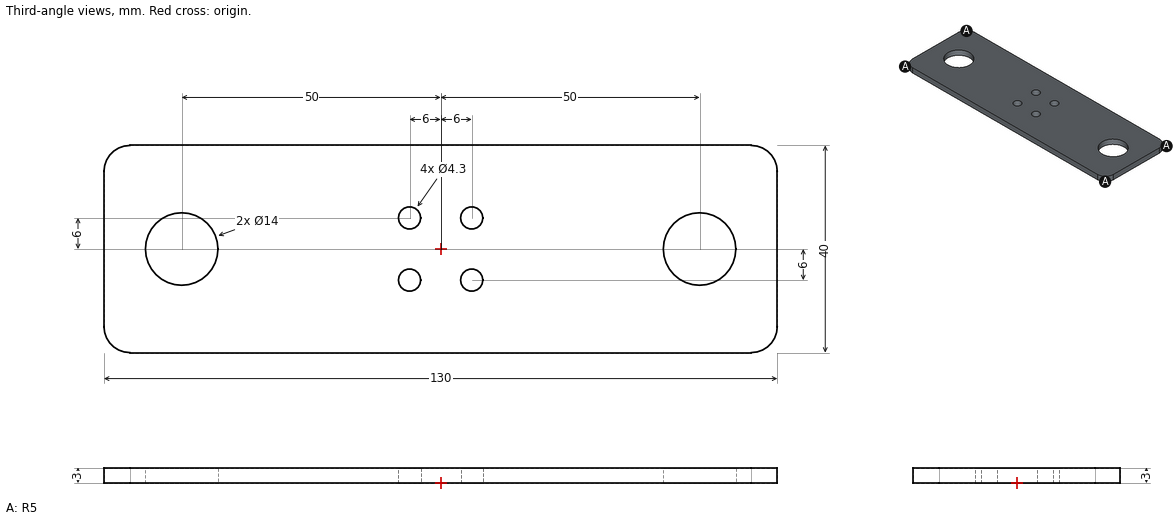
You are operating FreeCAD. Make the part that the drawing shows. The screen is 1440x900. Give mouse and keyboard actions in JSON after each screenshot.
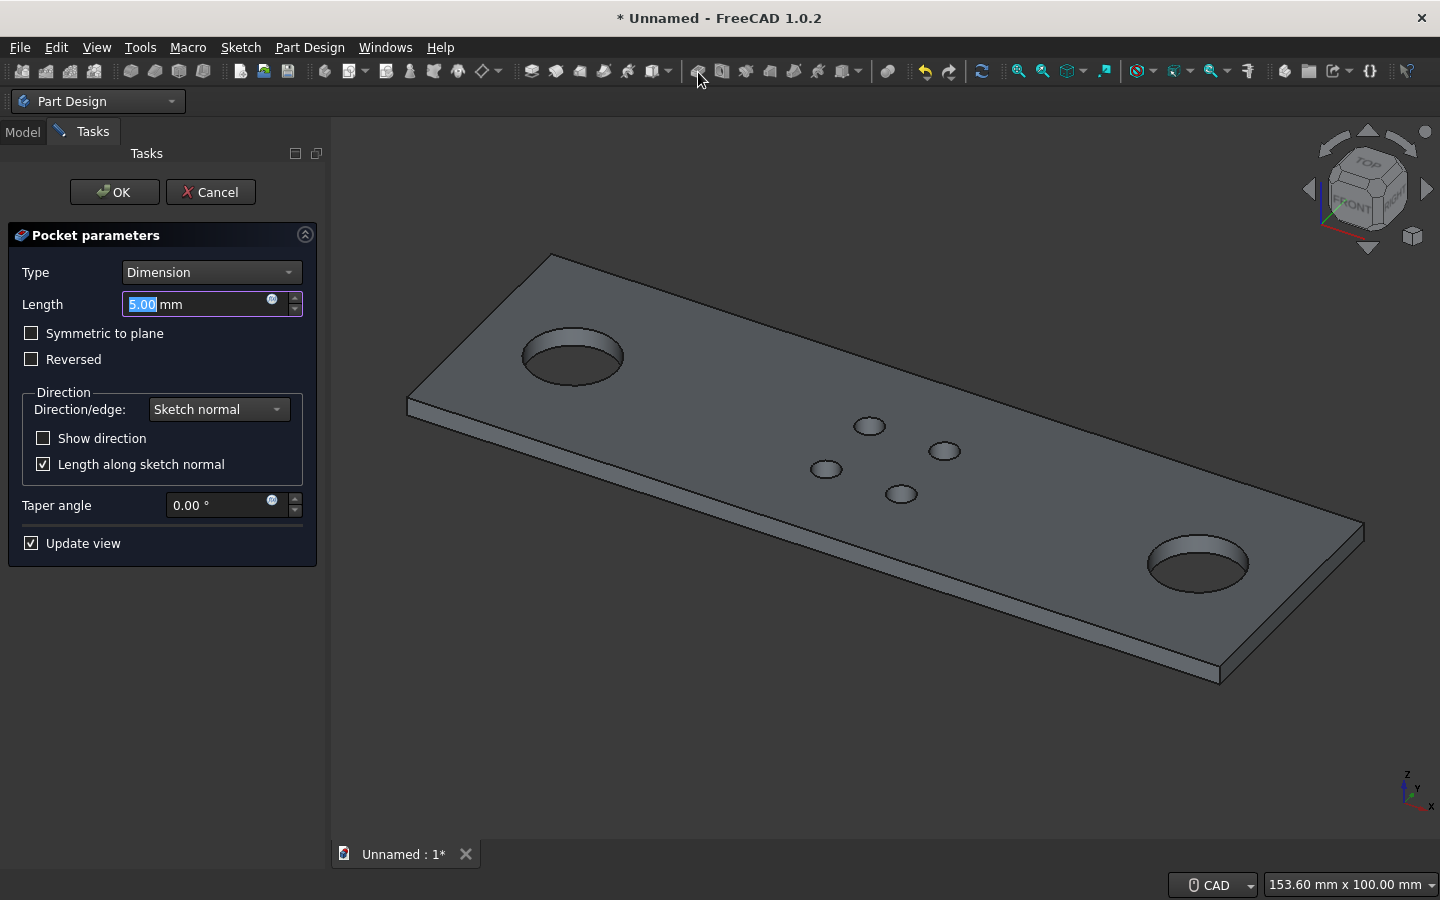
{"action": "type", "text": "3"}
{"action": "key", "text": "Tab"}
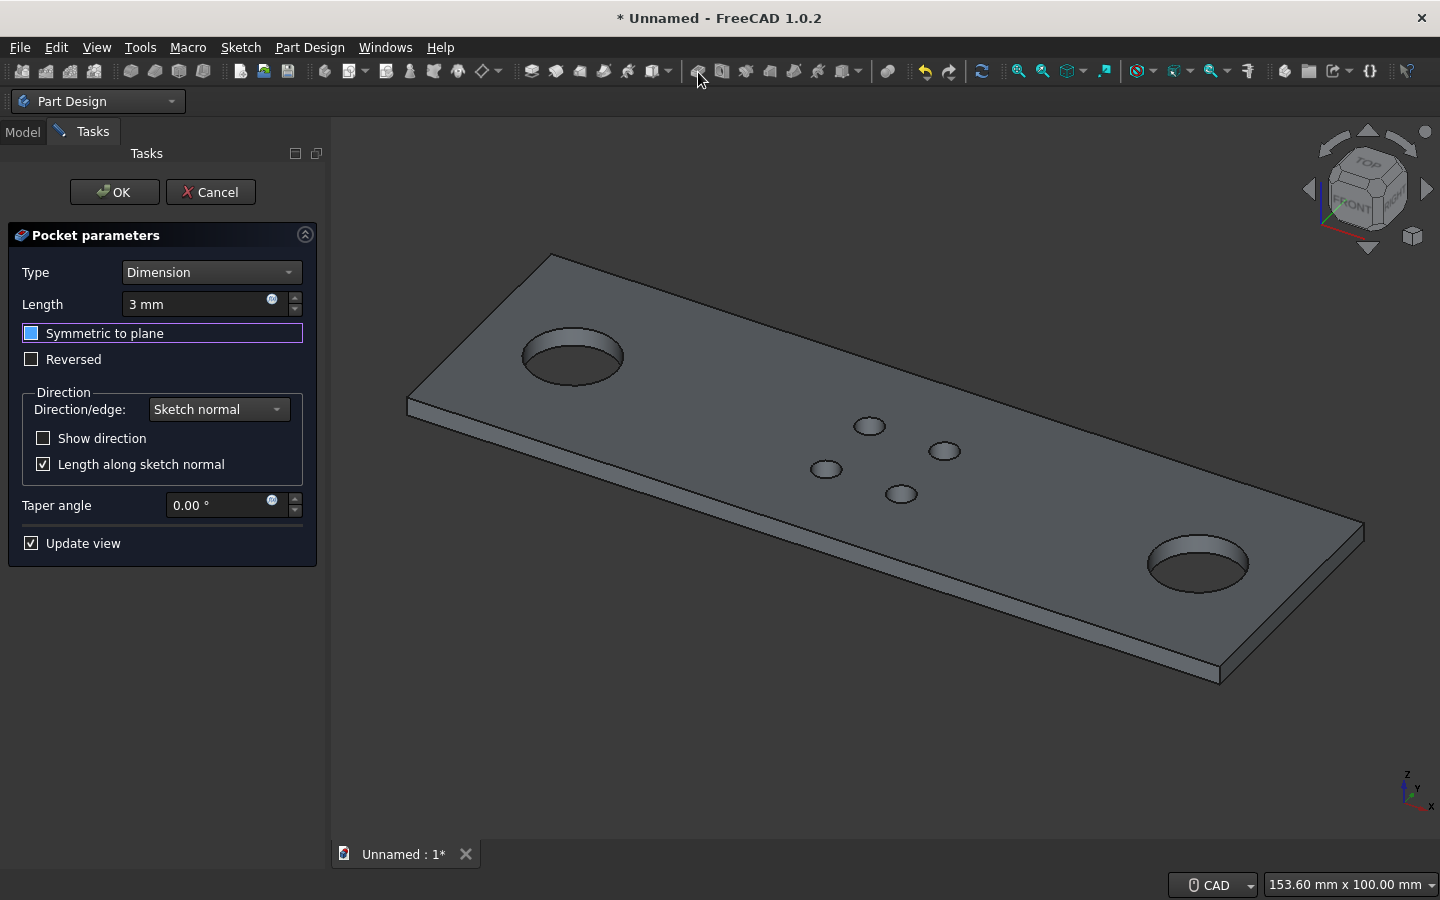
{"action": "left_click", "coordinate": [115, 192]}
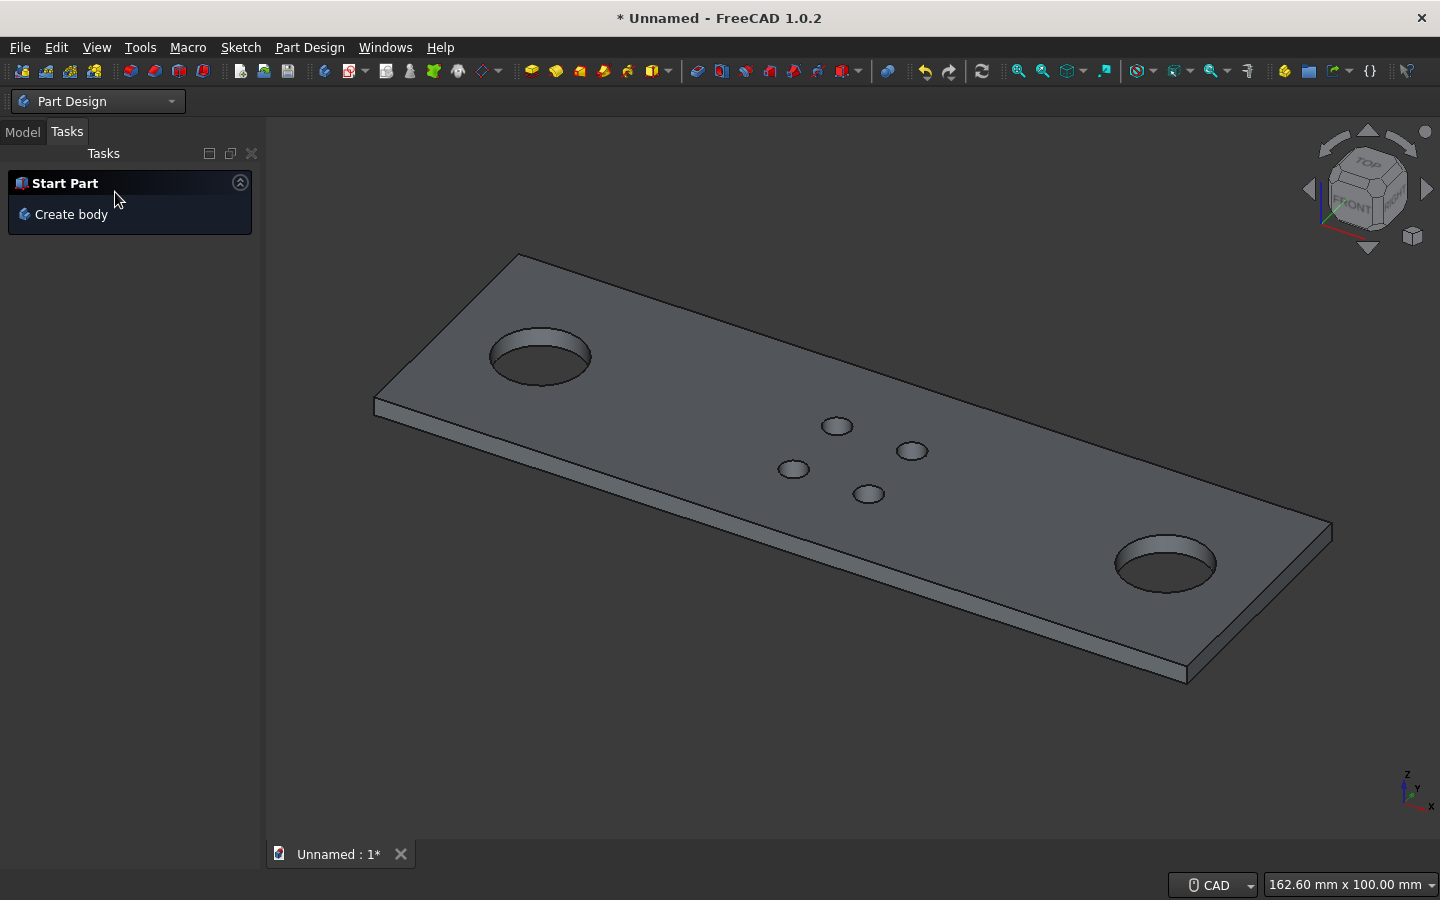
{"action": "left_click", "coordinate": [1187, 674]}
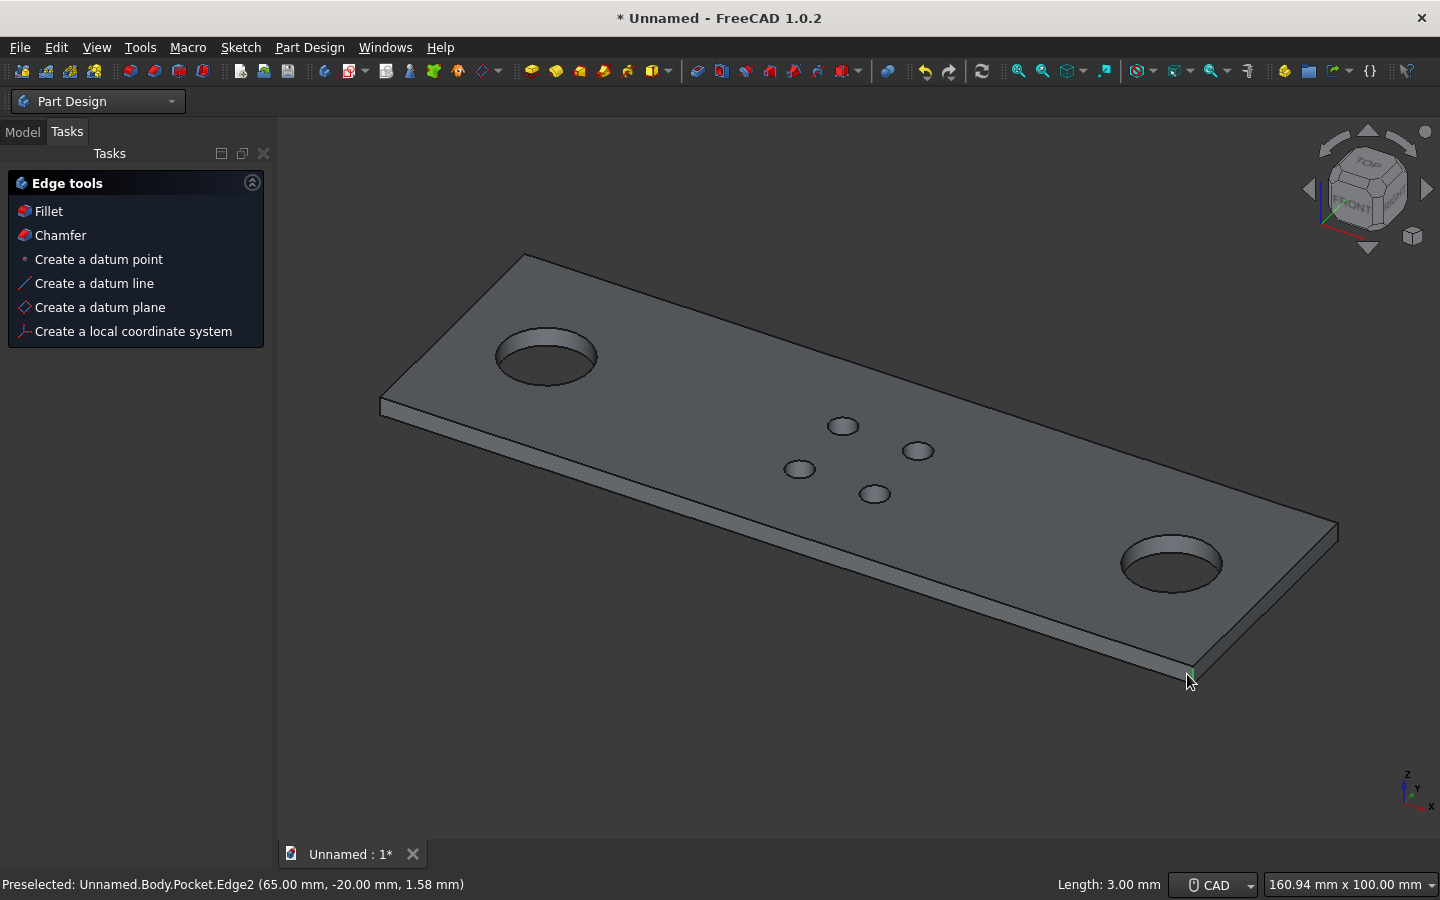
{"action": "scroll", "coordinate": [380, 405], "scroll_direction": "up", "scroll_amount": 4}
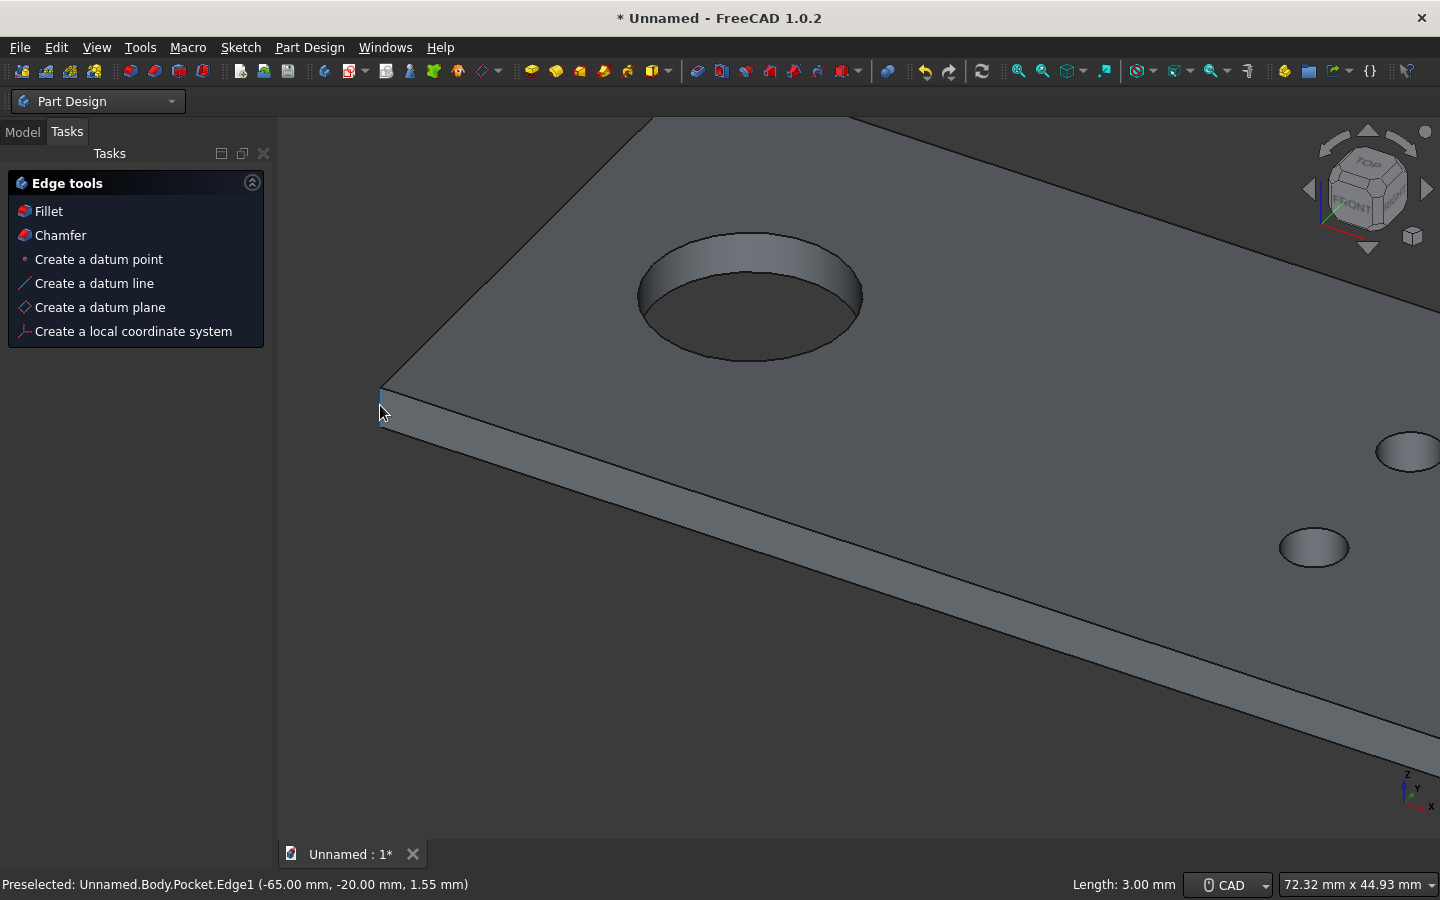
{"action": "left_click", "coordinate": [1020, 72]}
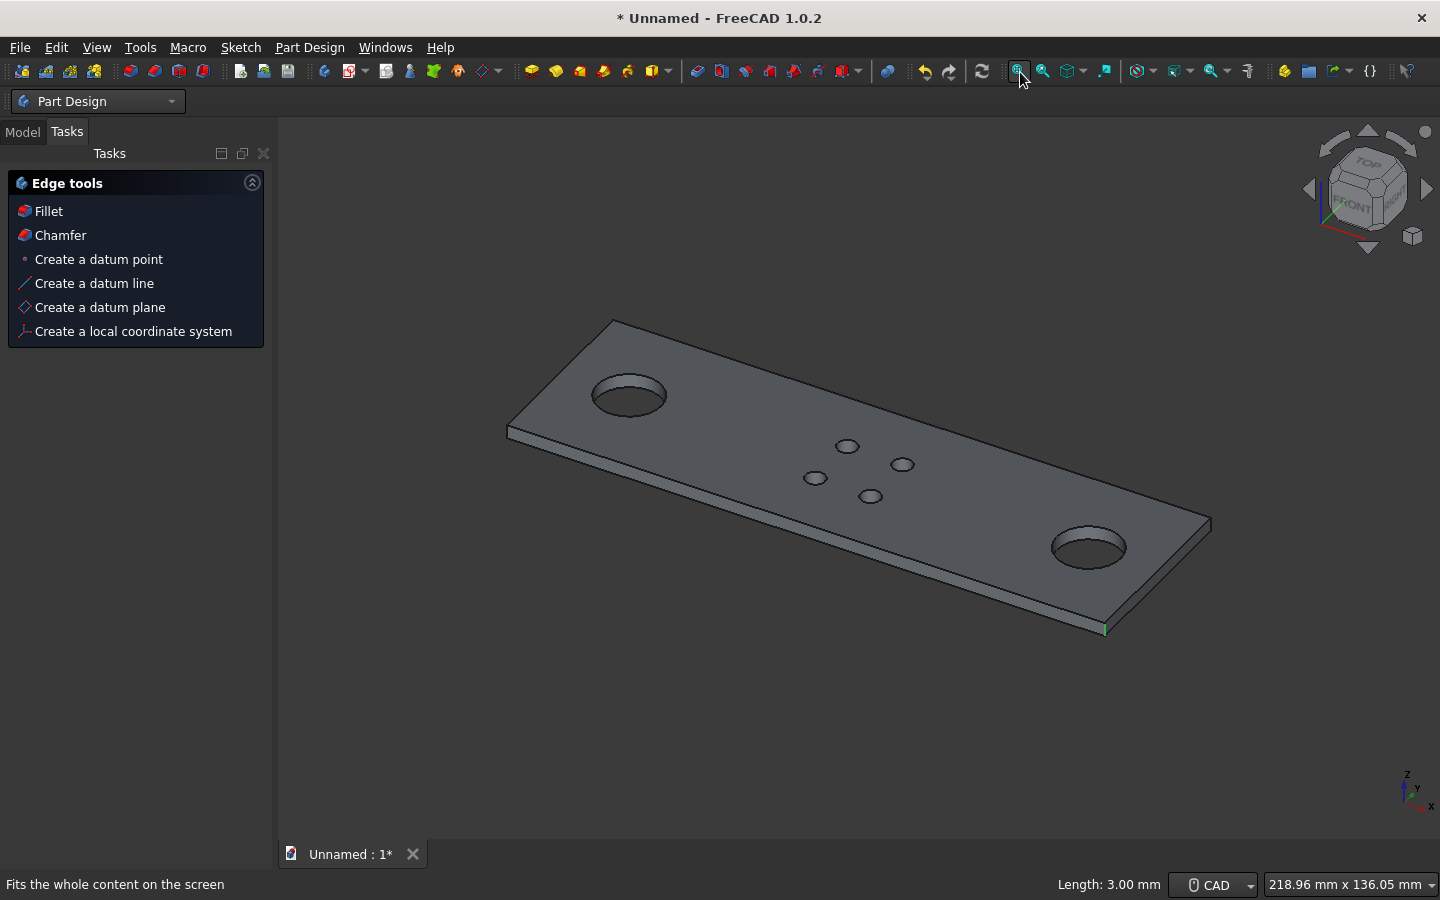
{"action": "key", "text": "0"}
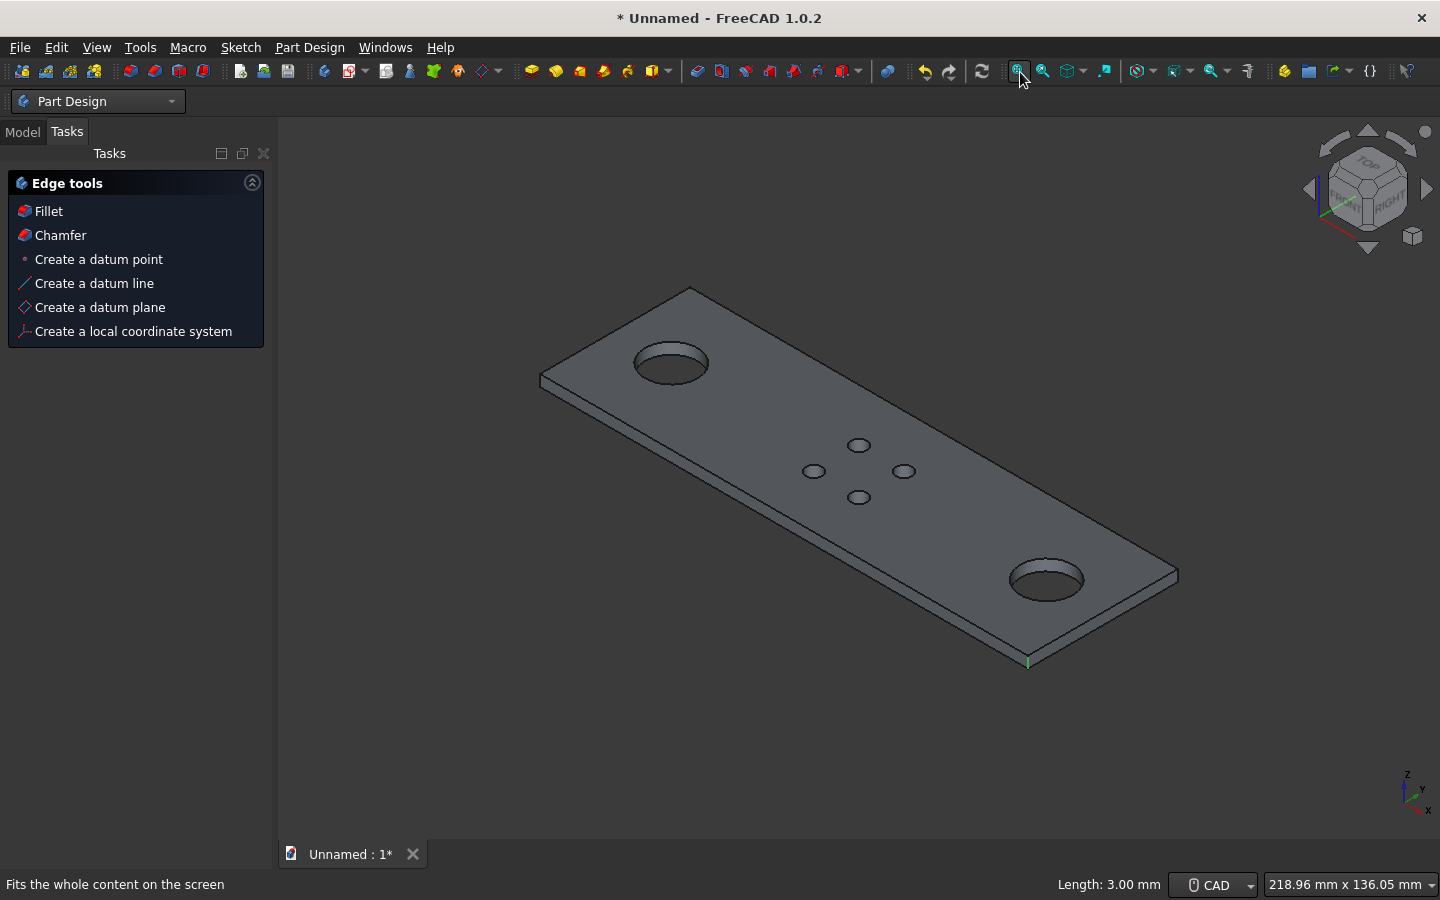
{"action": "scroll", "coordinate": [540, 380], "scroll_direction": "up", "scroll_amount": 5}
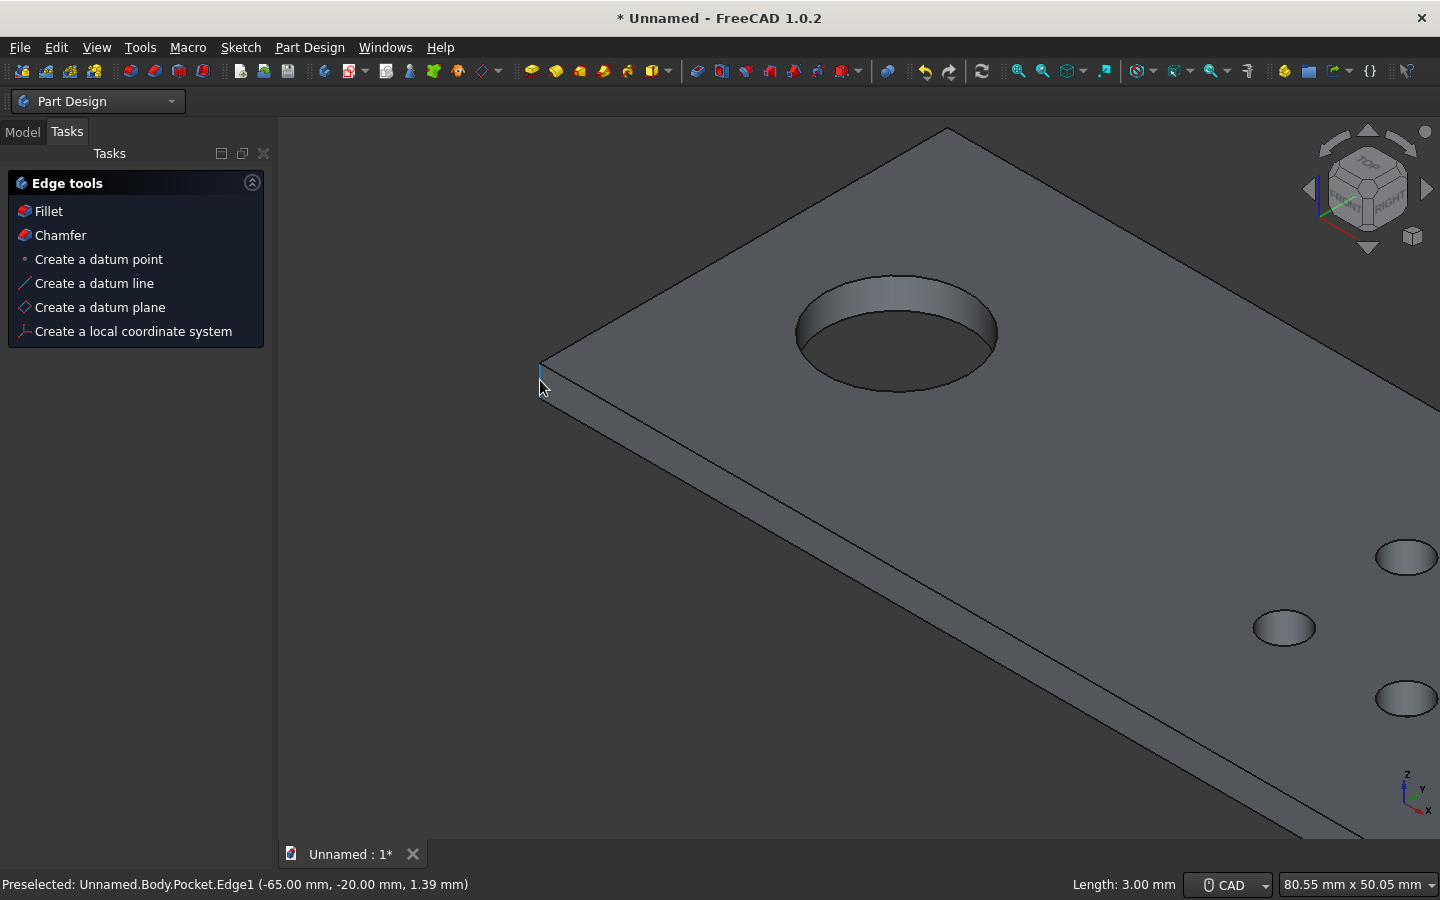
{"action": "key", "text": "v f"}